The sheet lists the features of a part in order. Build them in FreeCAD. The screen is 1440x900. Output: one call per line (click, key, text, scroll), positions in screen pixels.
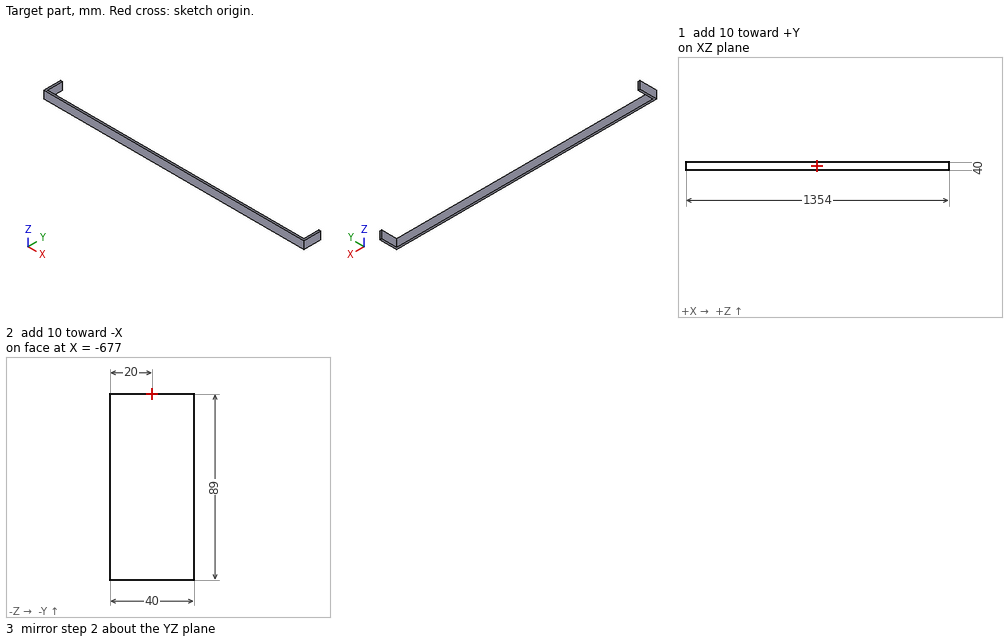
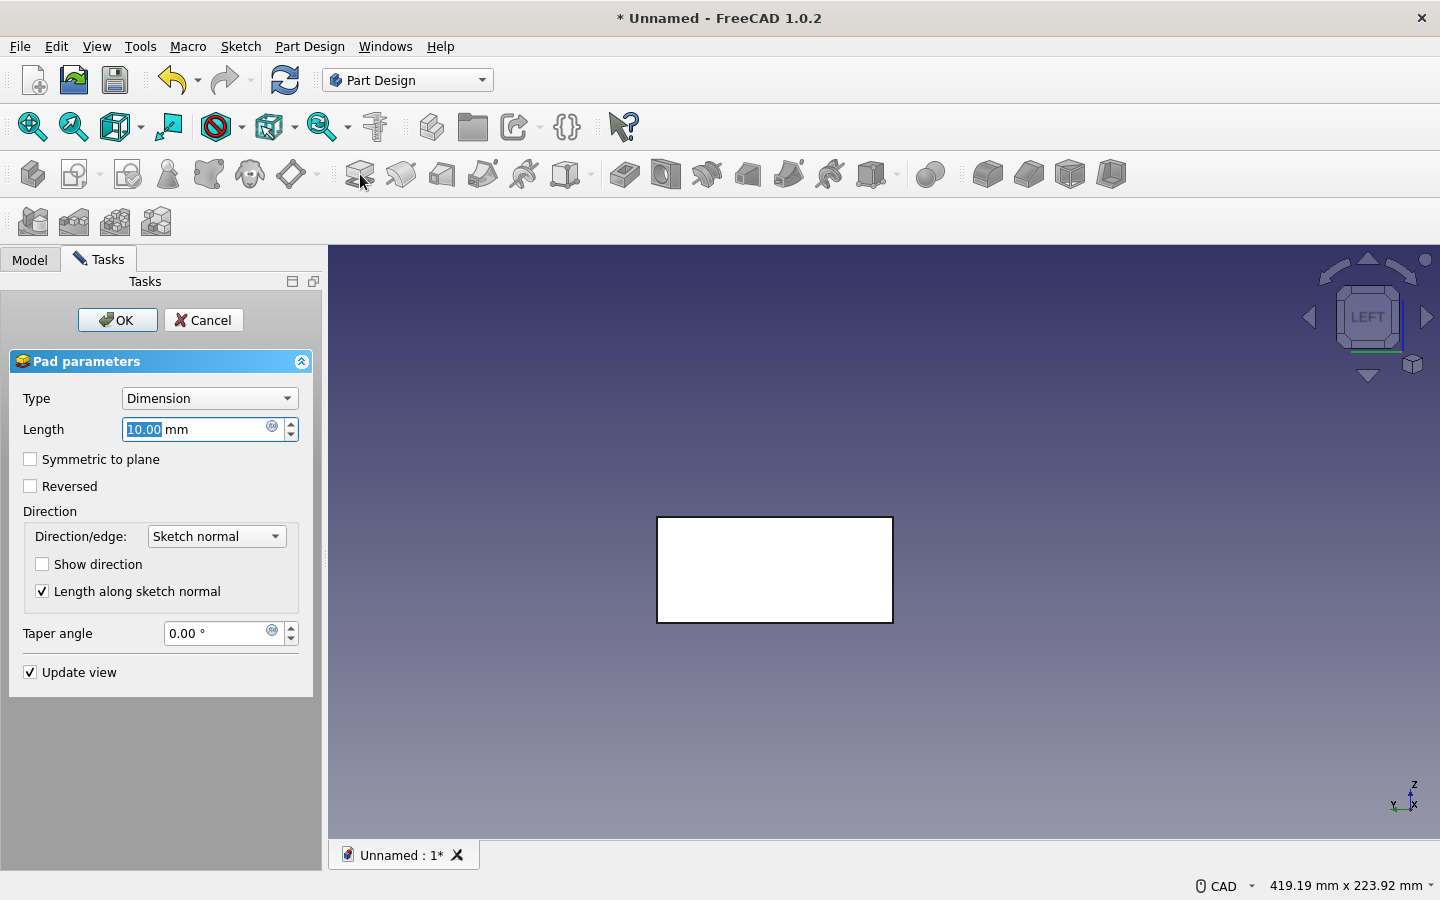
text(10)
key(Tab)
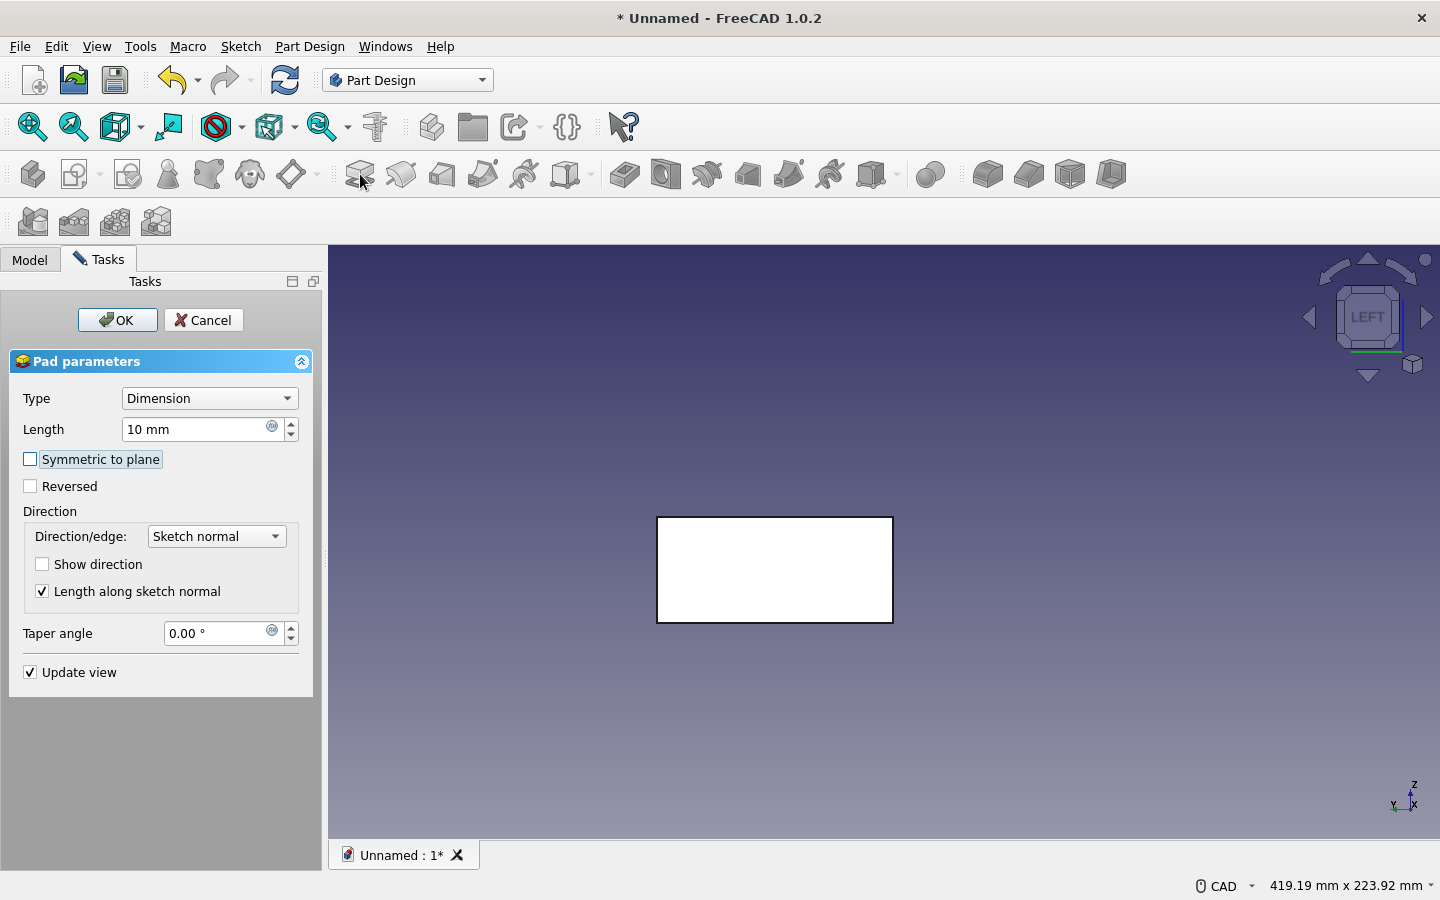
click(118, 320)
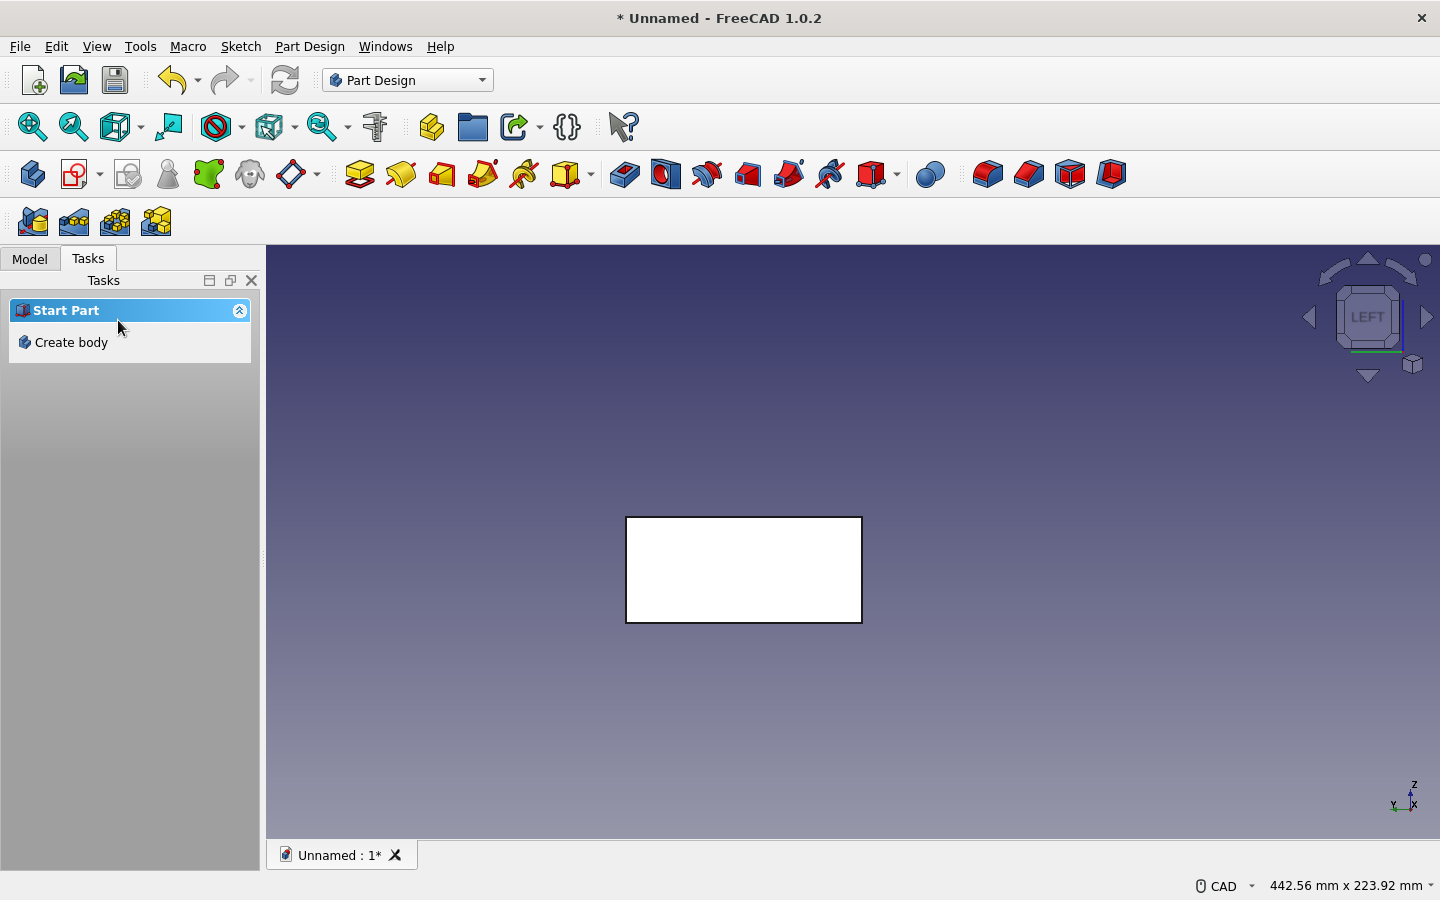
click(33, 128)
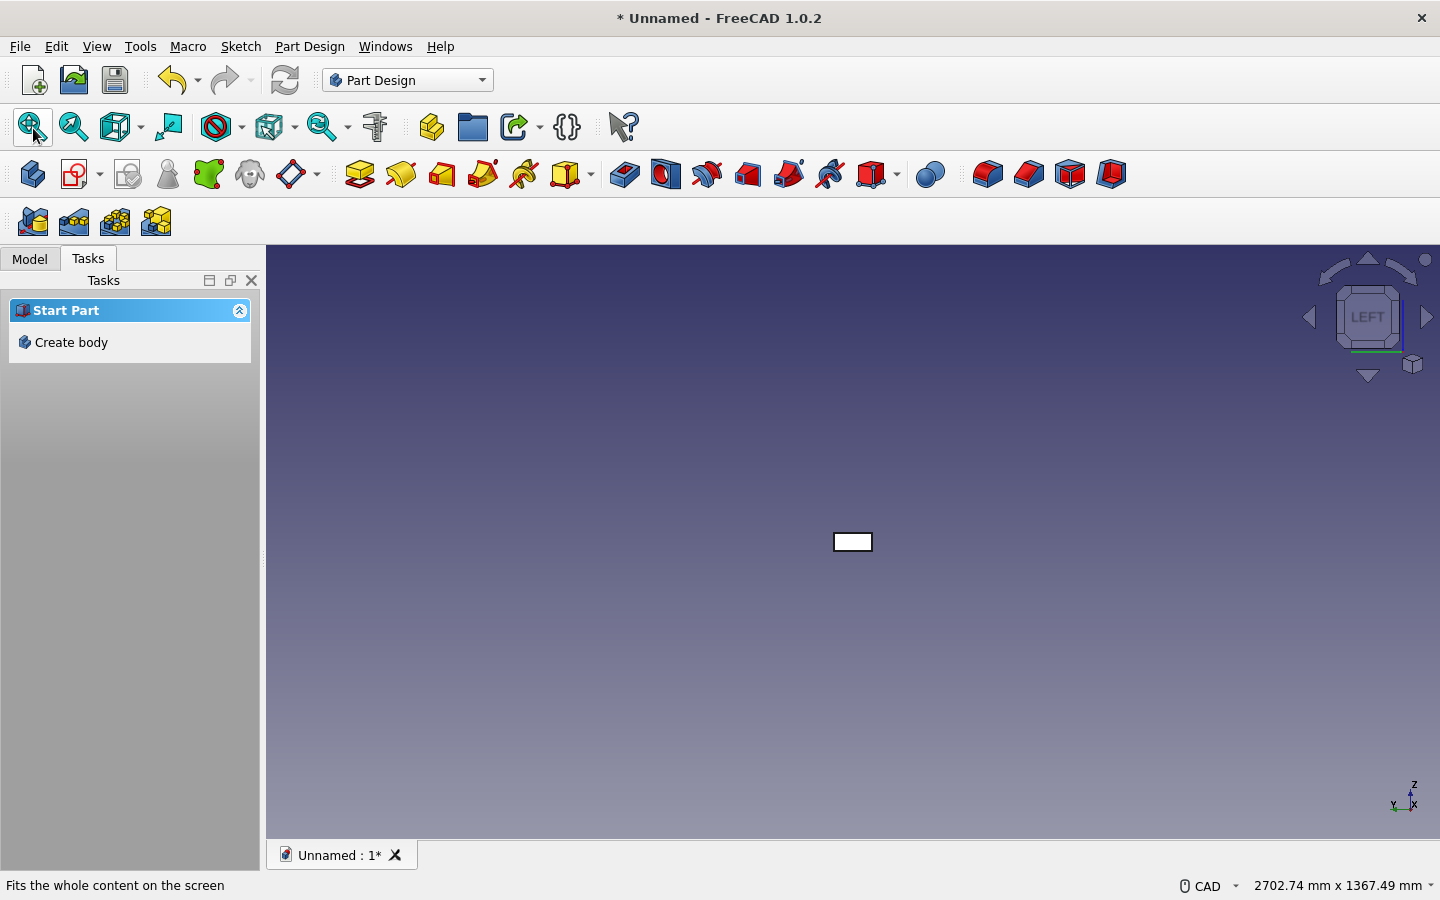
click(30, 258)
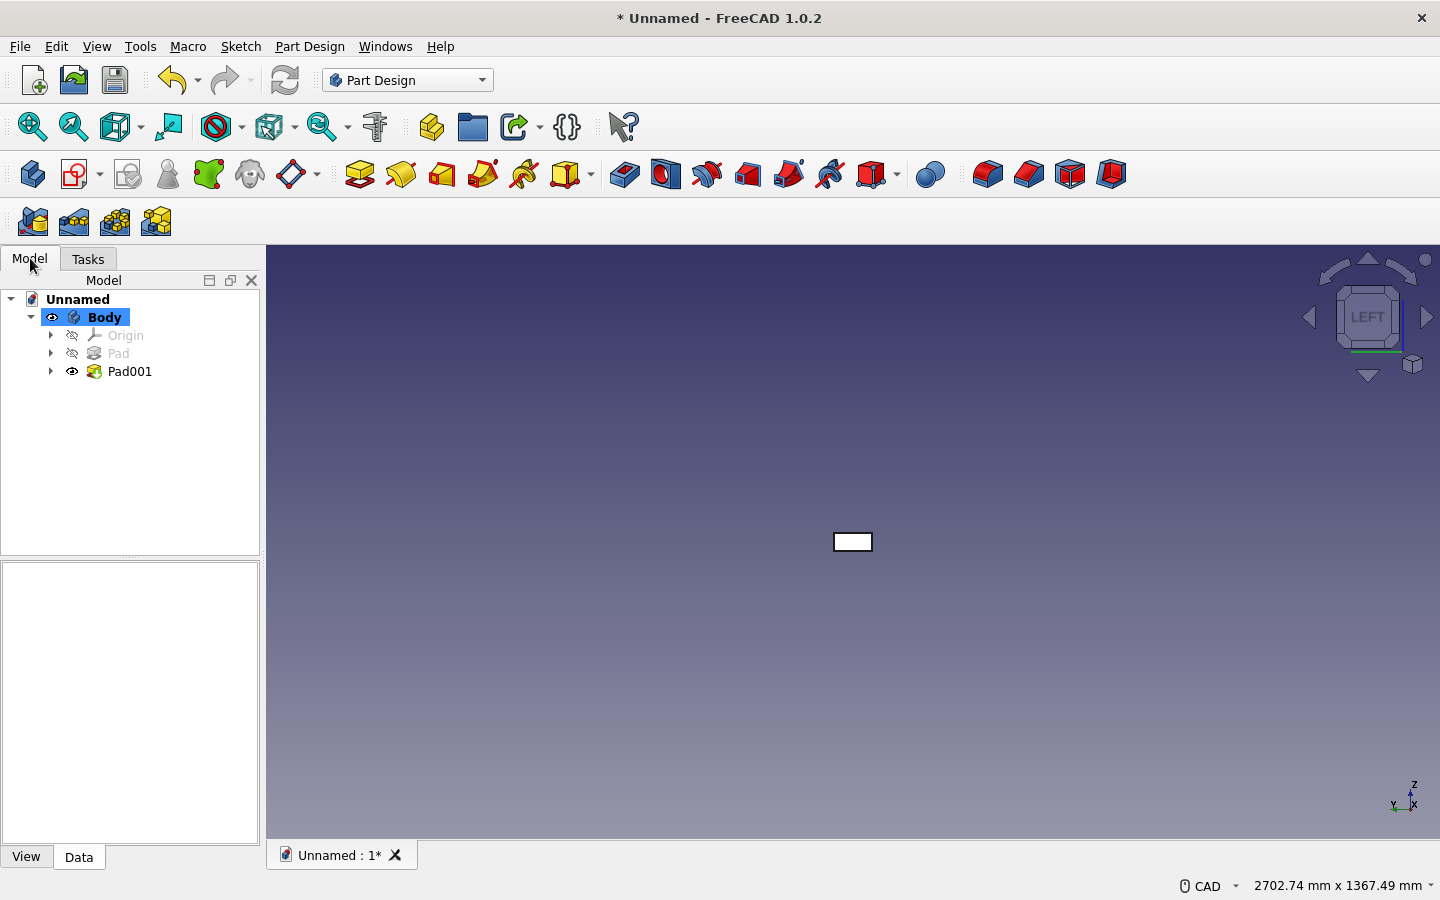
click(117, 371)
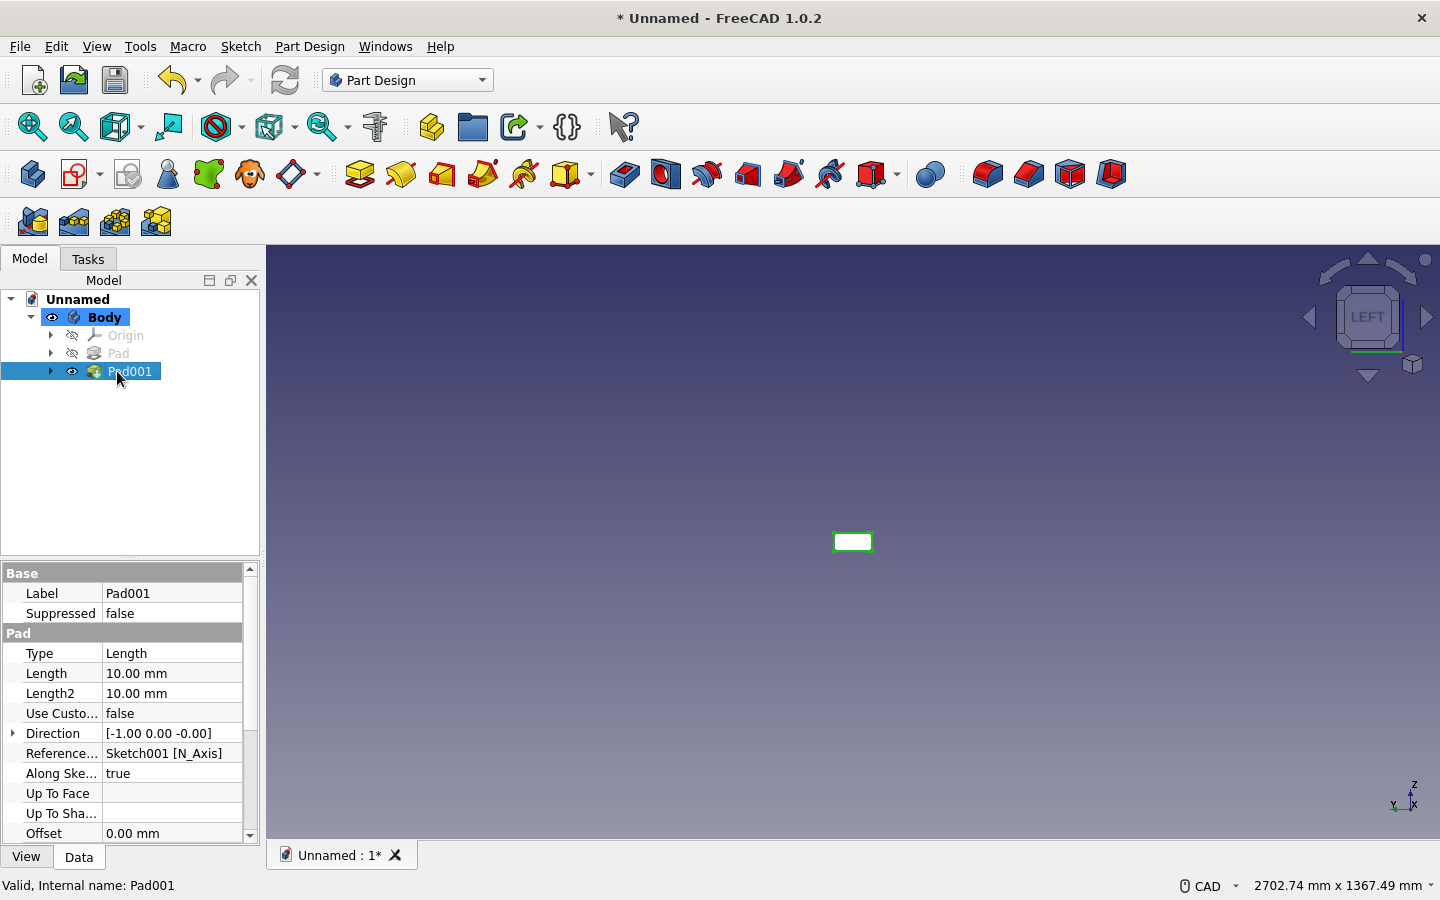
click(33, 222)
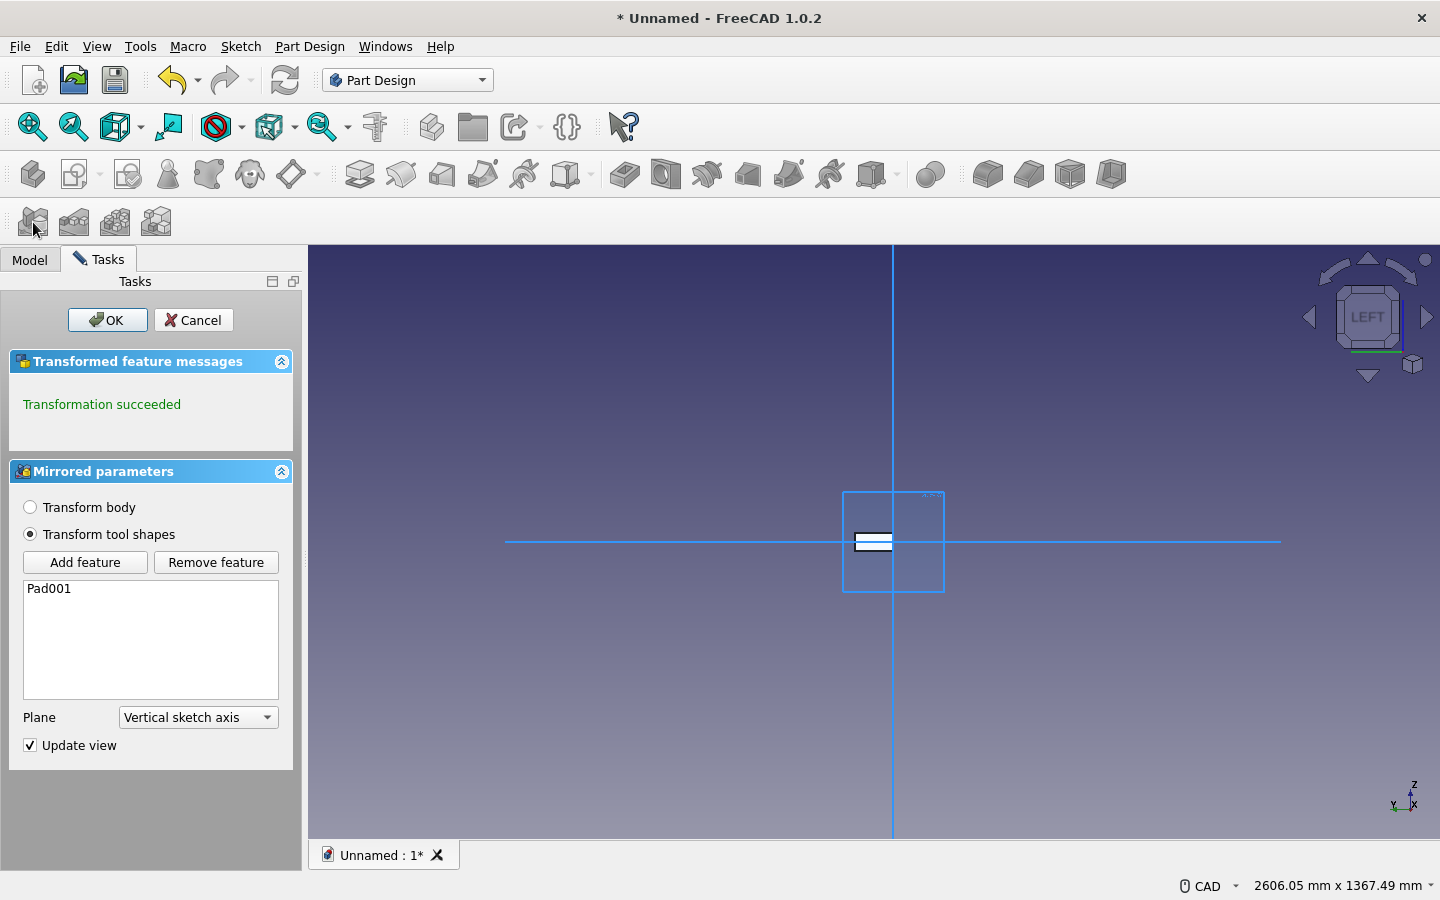
click(199, 718)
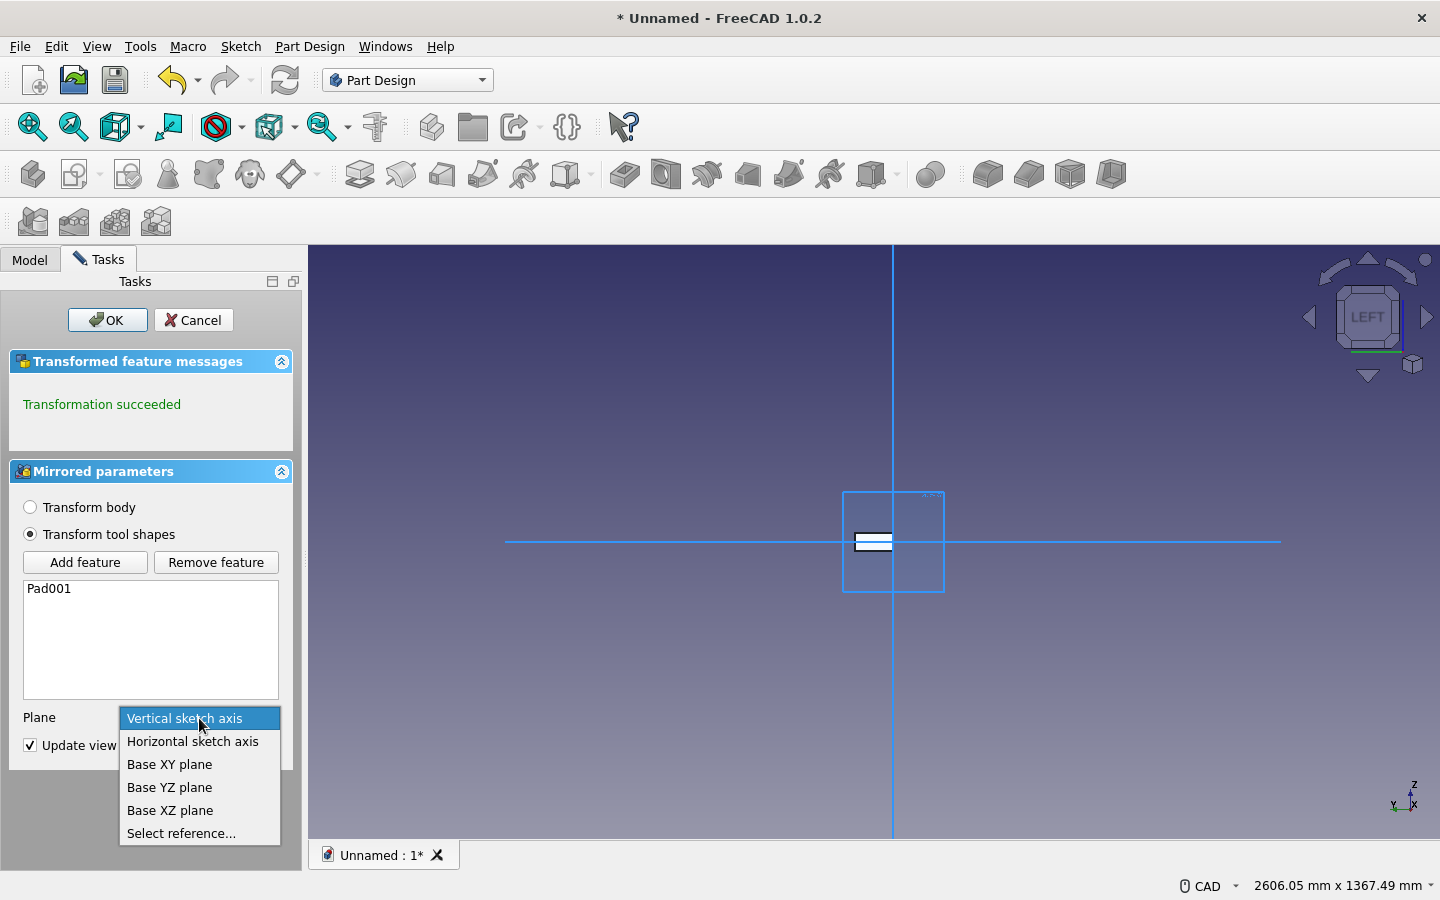
click(198, 788)